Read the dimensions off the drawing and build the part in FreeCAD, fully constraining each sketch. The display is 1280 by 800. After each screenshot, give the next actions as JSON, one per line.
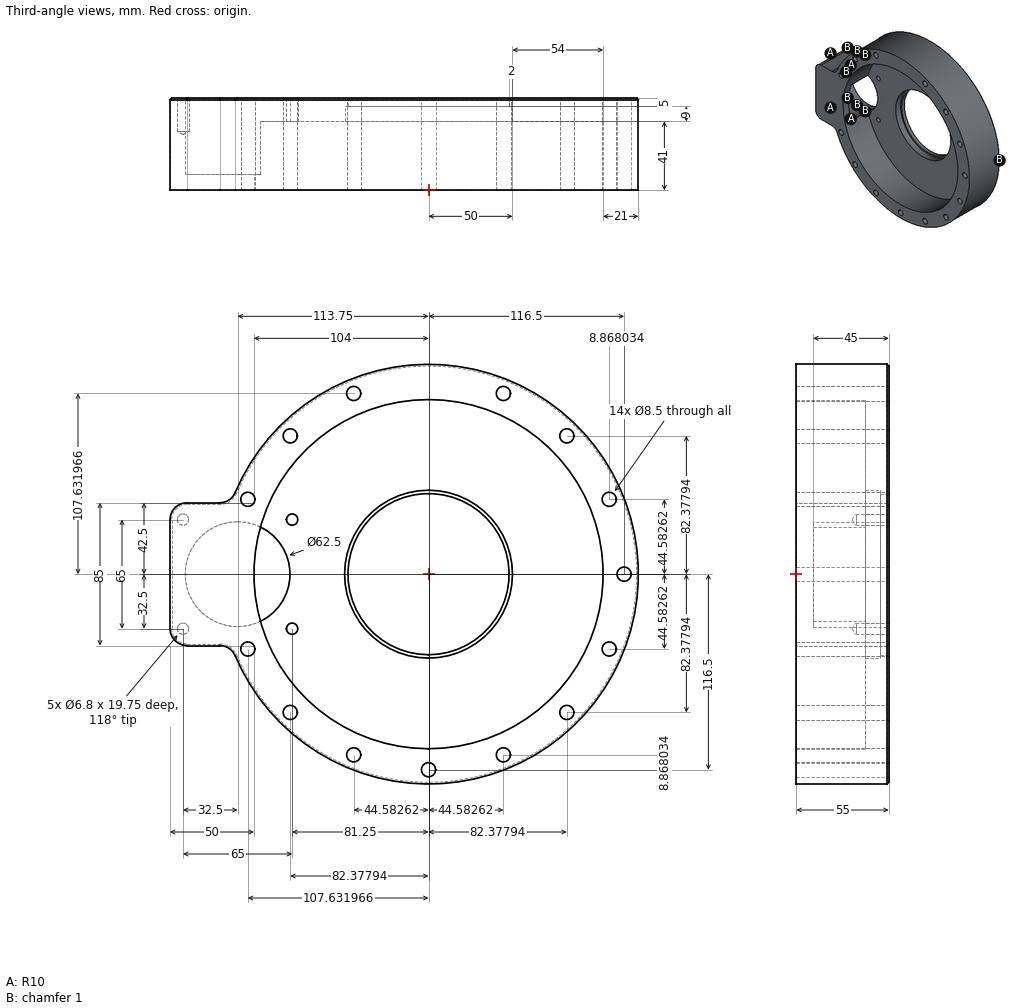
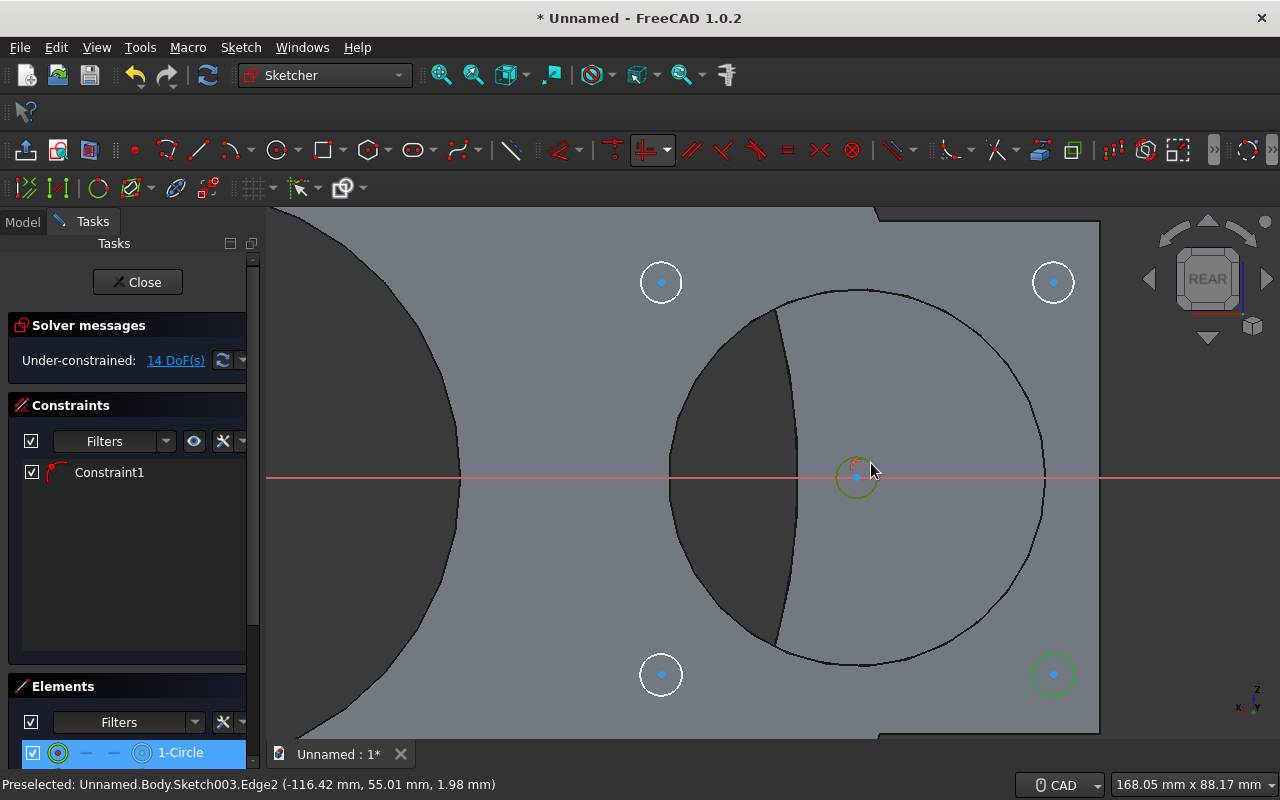
{"action": "left_click", "coordinate": [676, 660]}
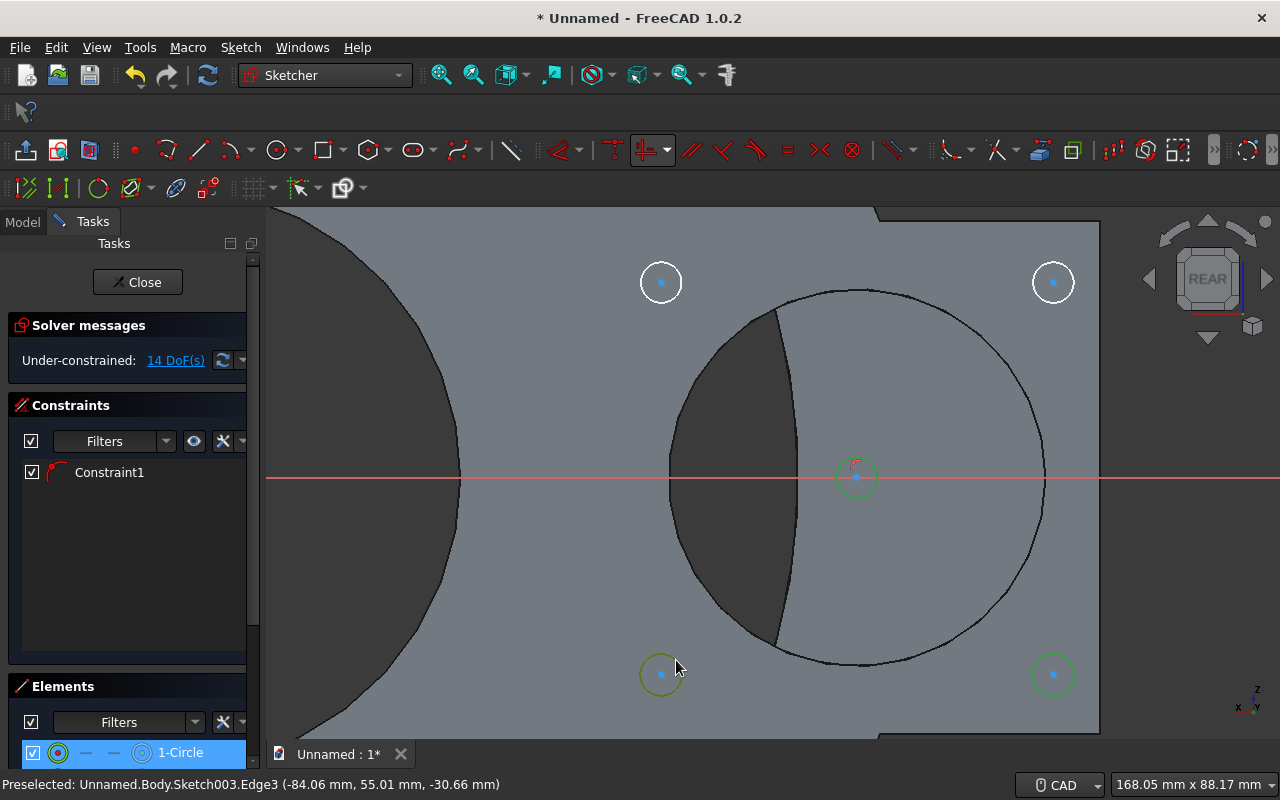
{"action": "left_click", "coordinate": [1068, 268]}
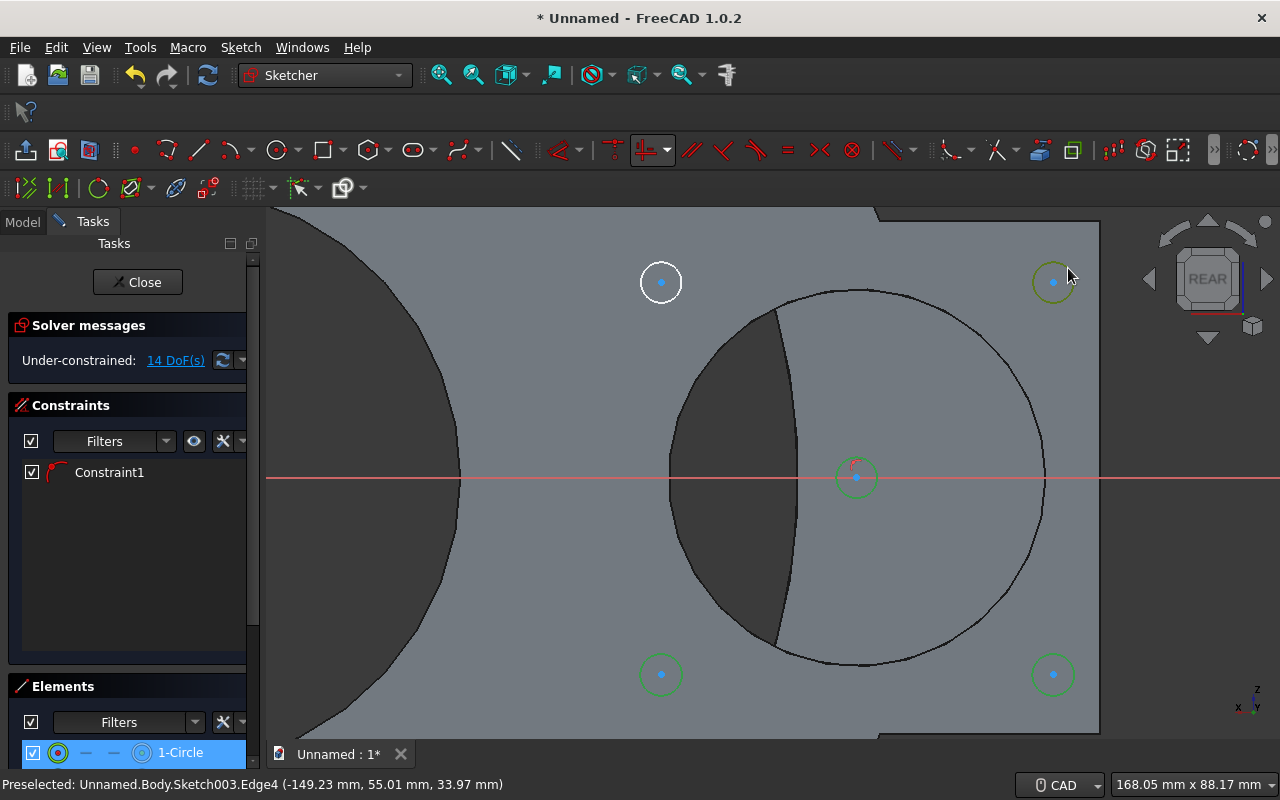
{"action": "left_click", "coordinate": [675, 268]}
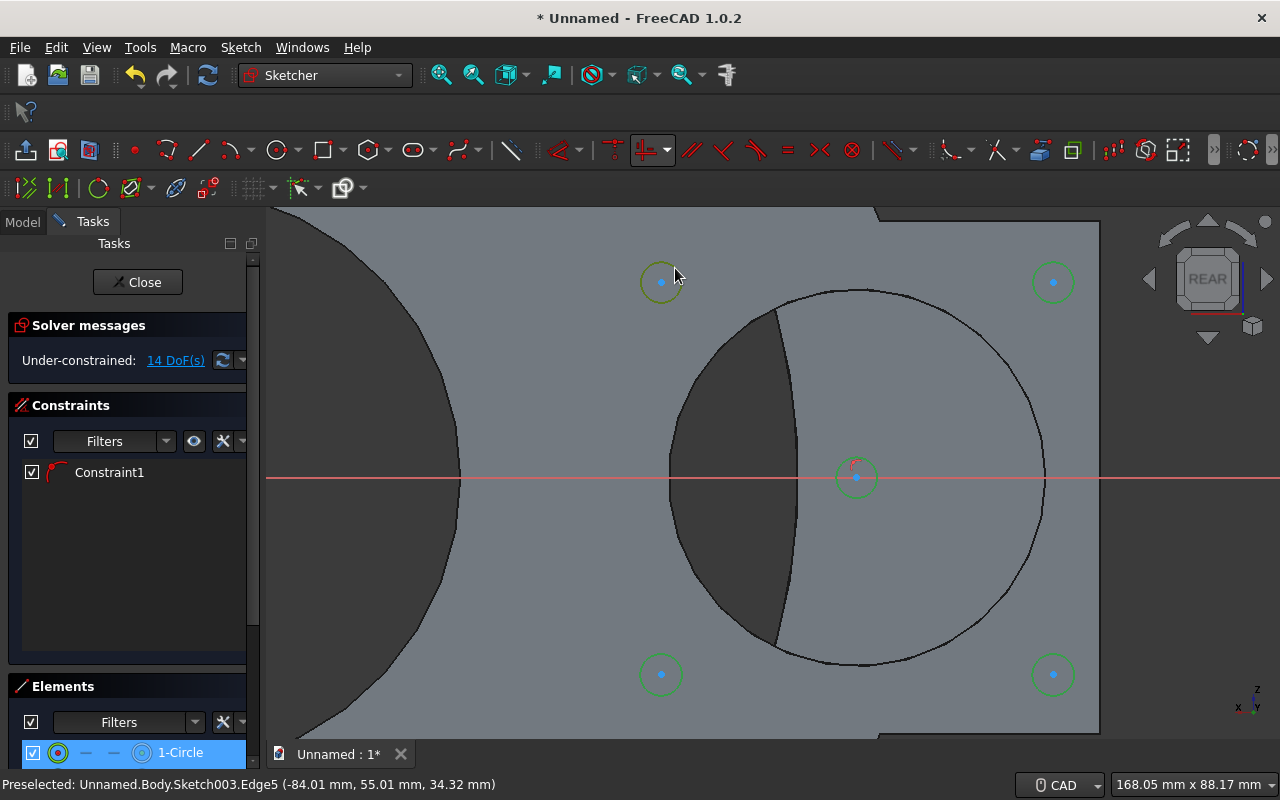
{"action": "left_click", "coordinate": [788, 150]}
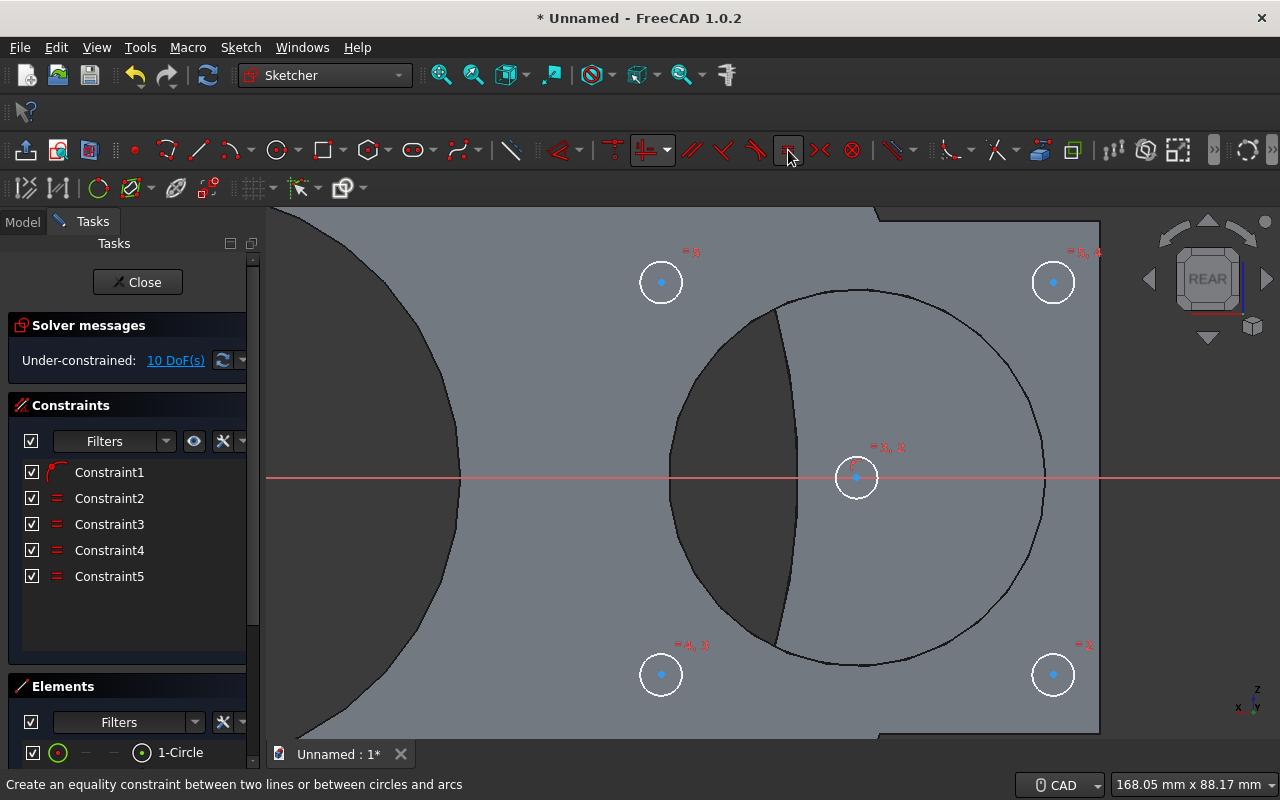
{"action": "left_click", "coordinate": [1053, 675]}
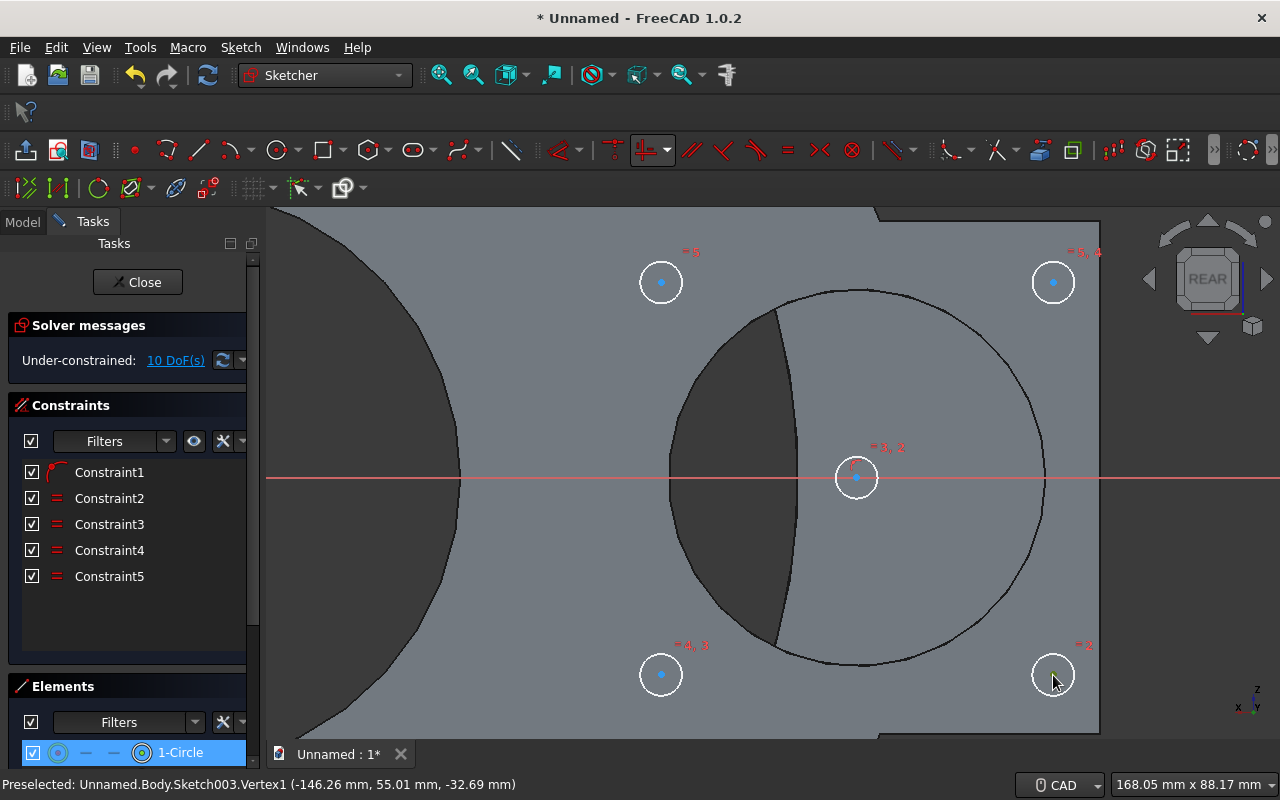
{"action": "left_click", "coordinate": [661, 675]}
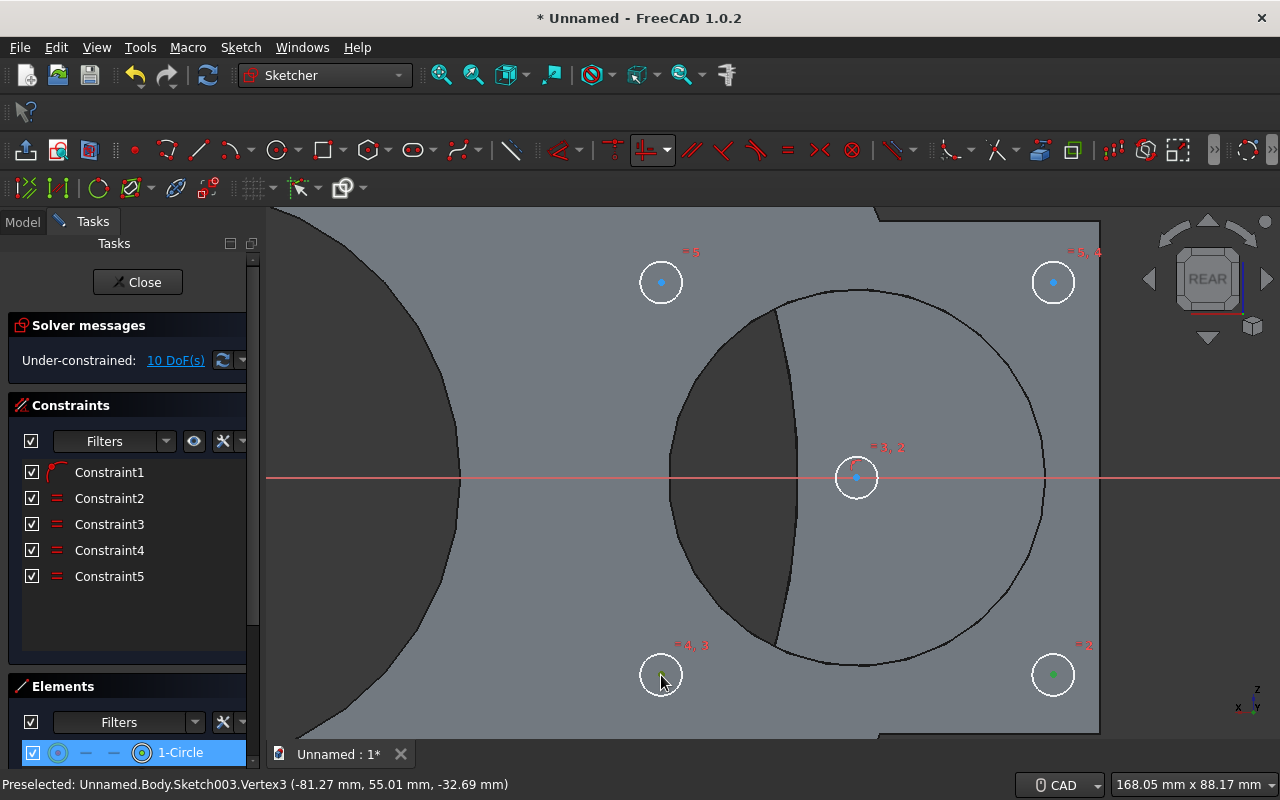
{"action": "key", "text": "h"}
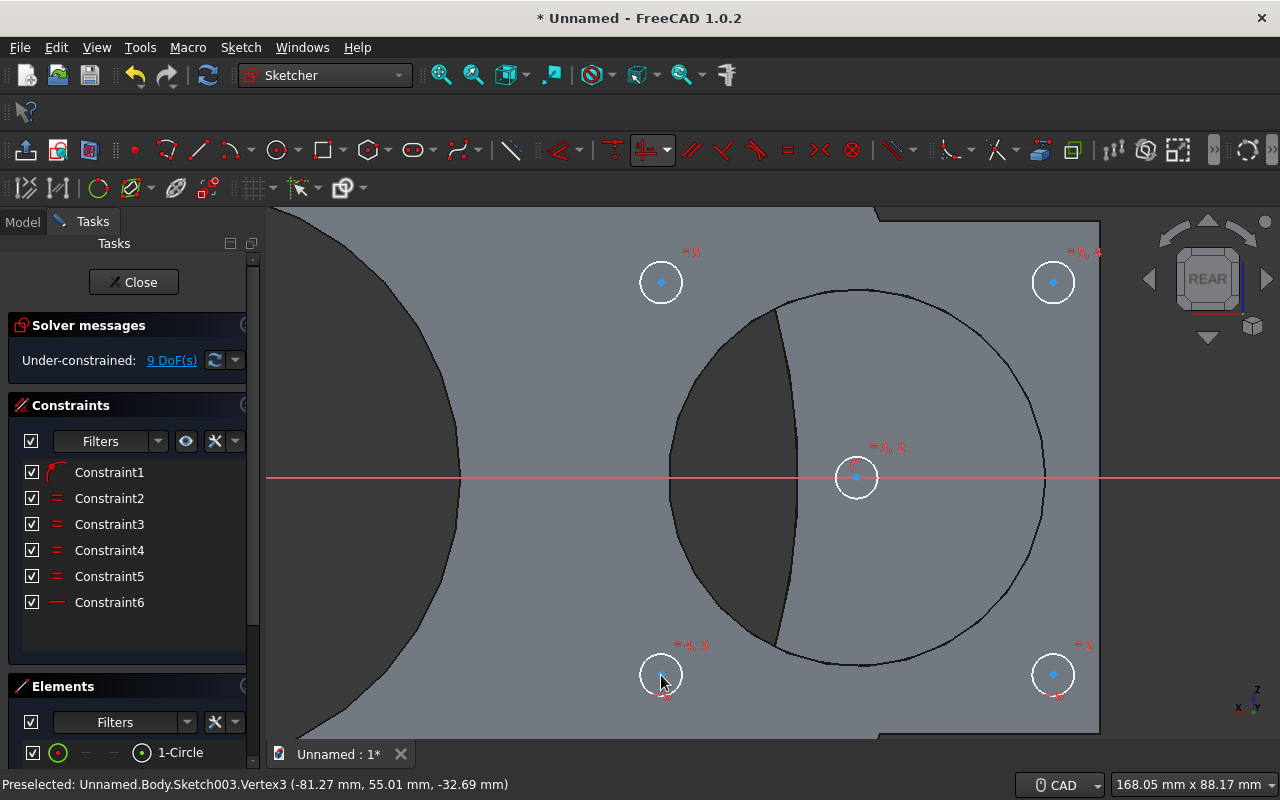
{"action": "left_click", "coordinate": [1053, 675]}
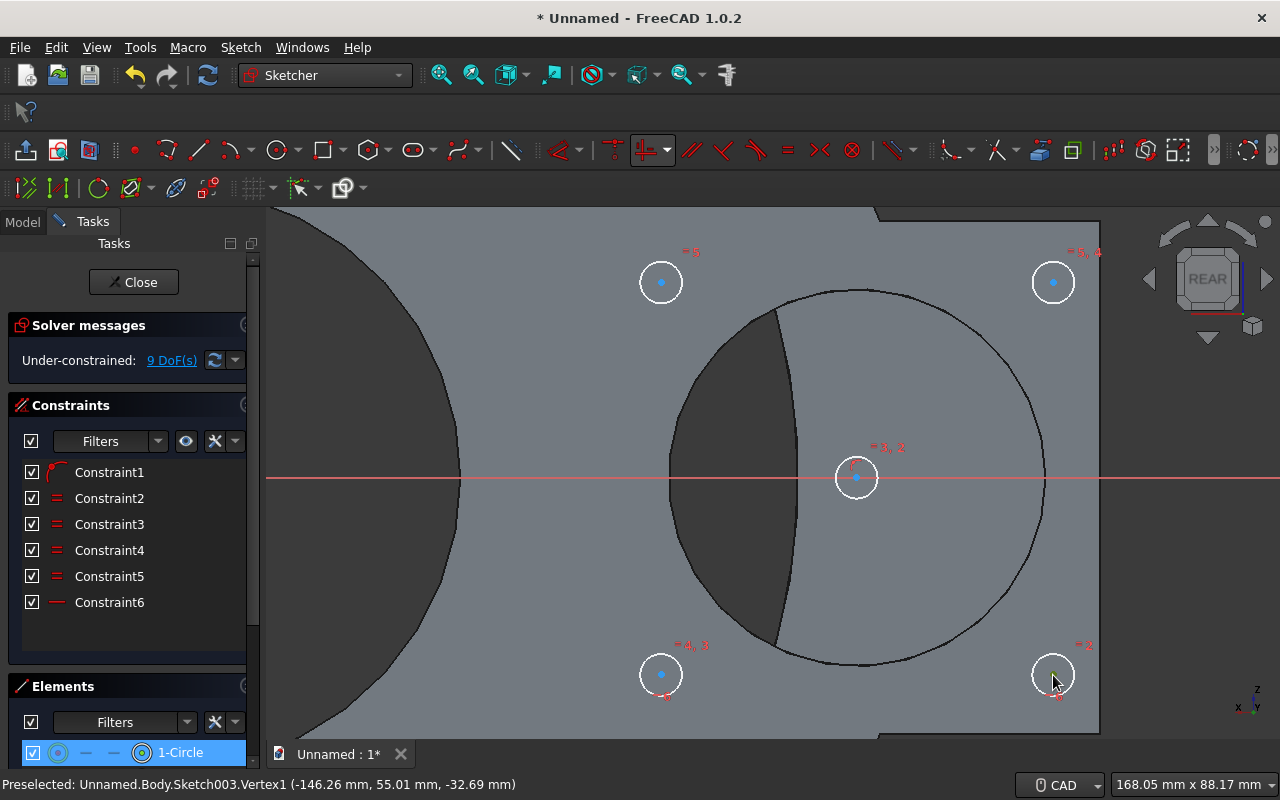
{"action": "left_click", "coordinate": [1053, 283]}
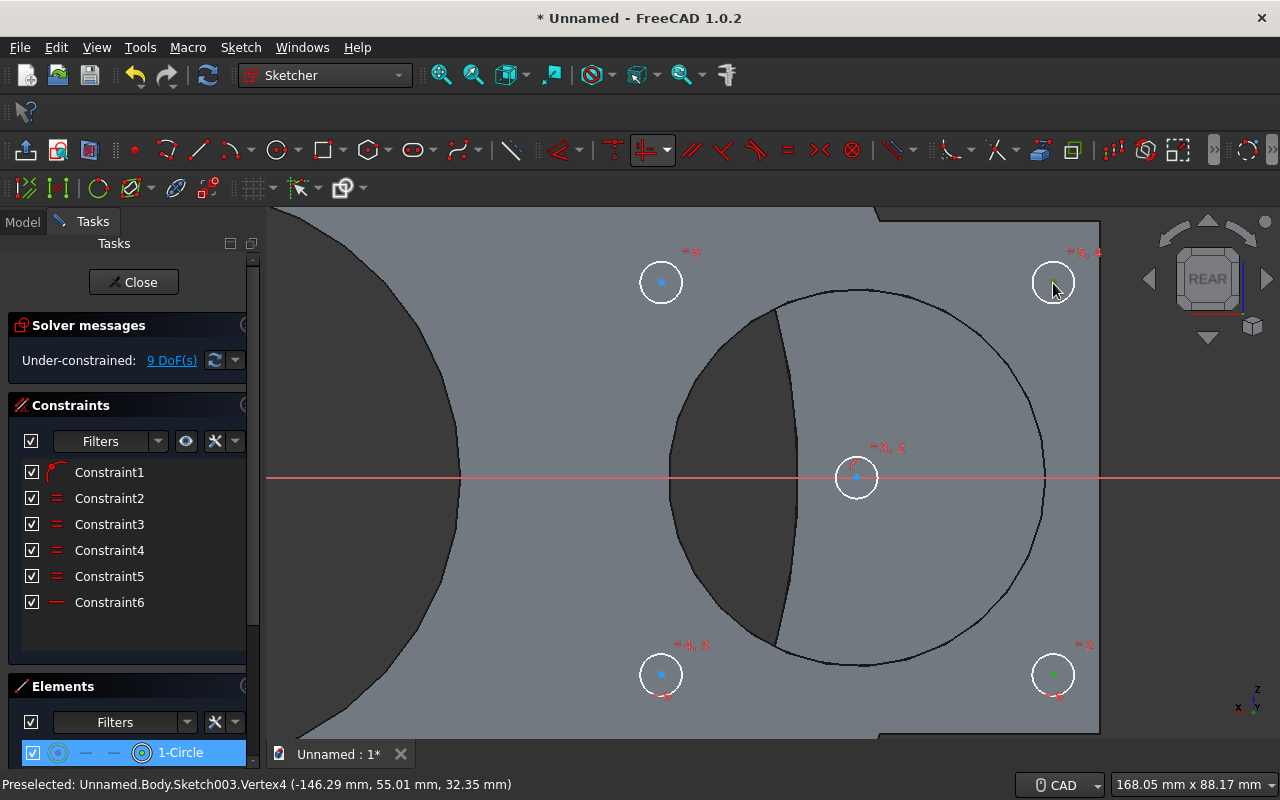
{"action": "left_click", "coordinate": [670, 150]}